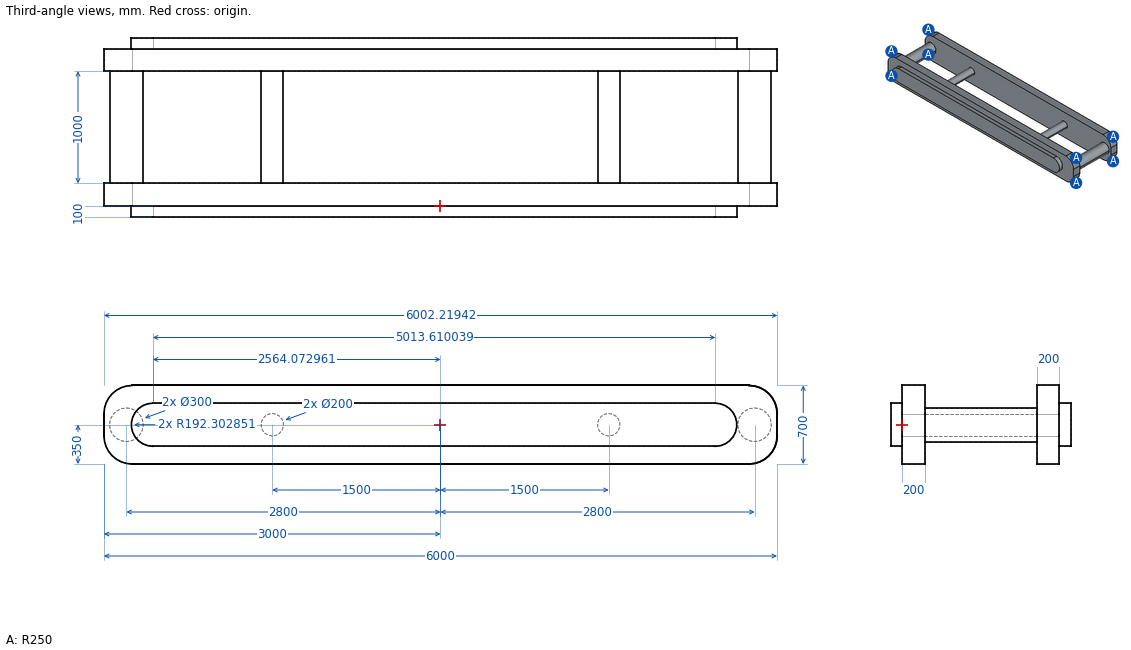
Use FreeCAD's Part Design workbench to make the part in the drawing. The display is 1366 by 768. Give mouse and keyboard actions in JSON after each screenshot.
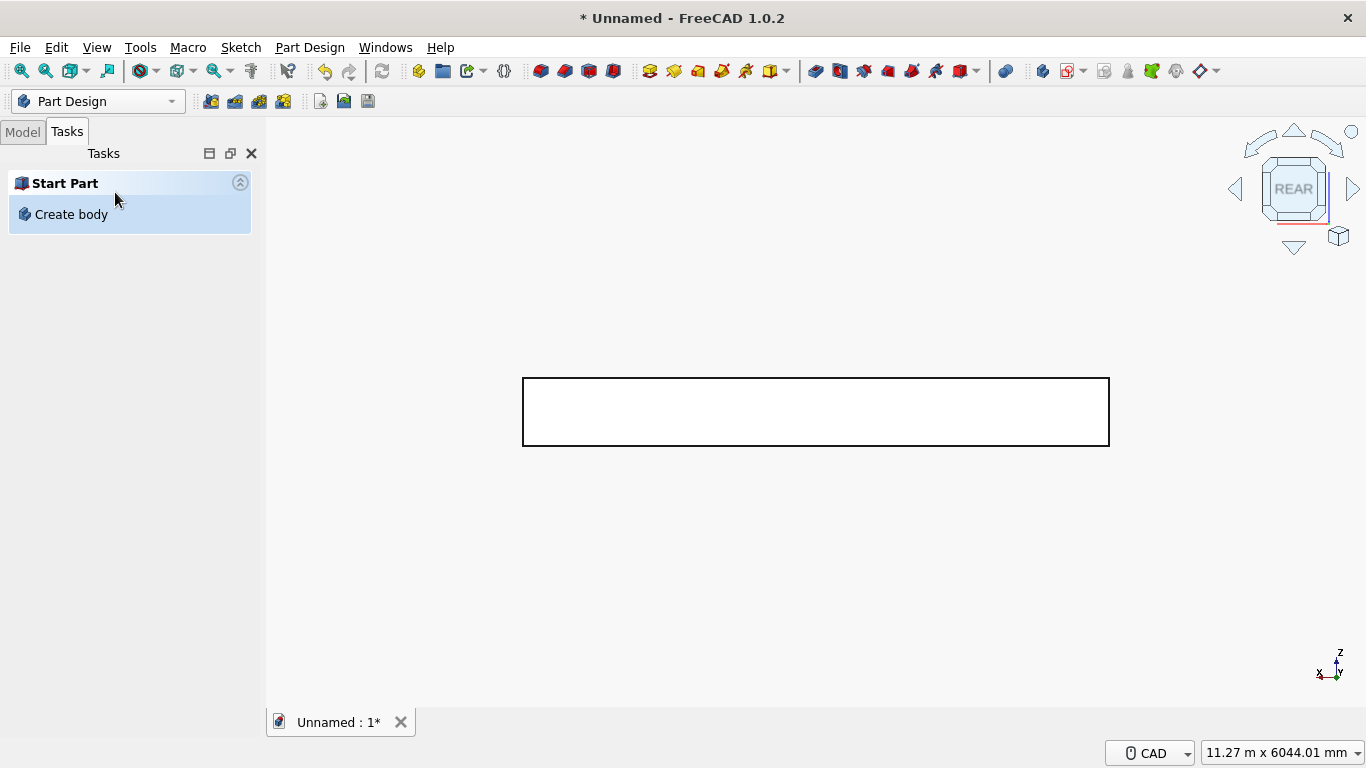
{"action": "scroll", "coordinate": [523, 445], "scroll_direction": "up", "scroll_amount": 4}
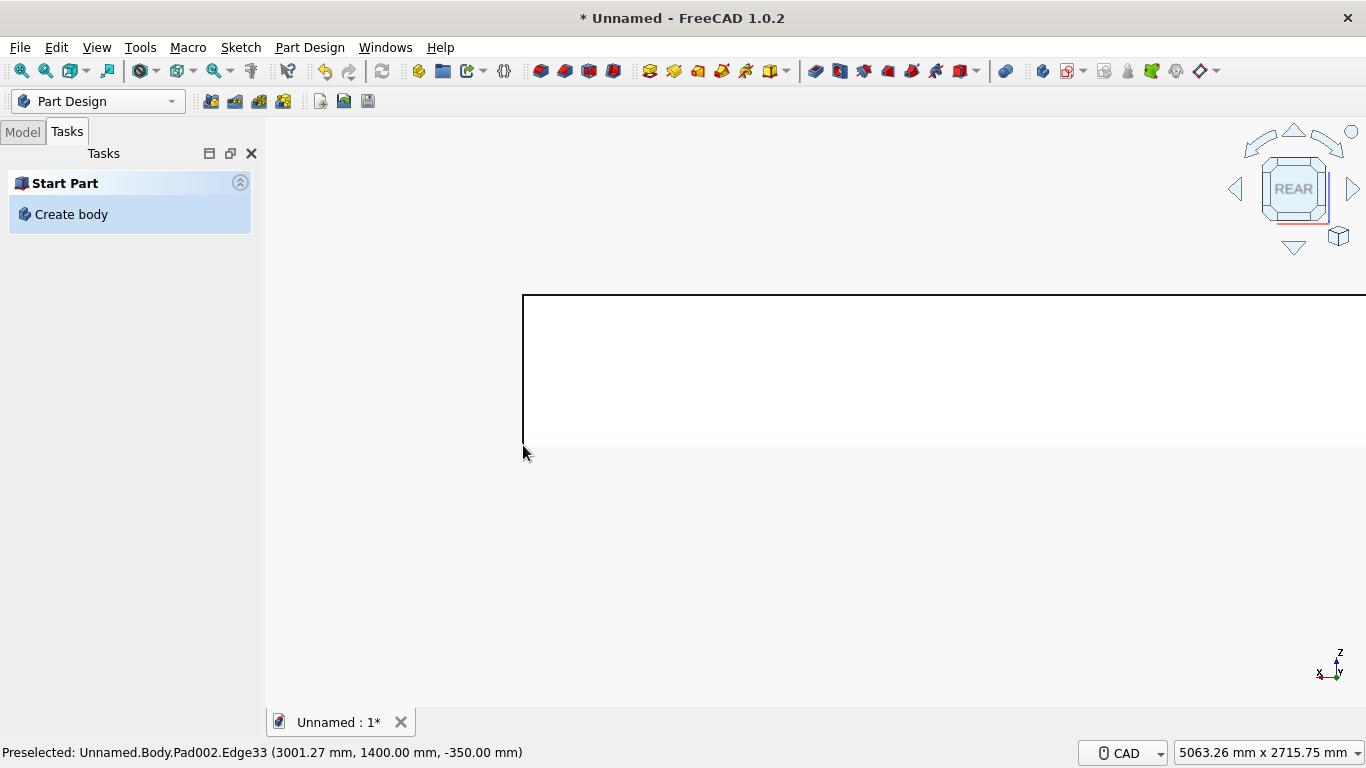
{"action": "left_click", "coordinate": [22, 72]}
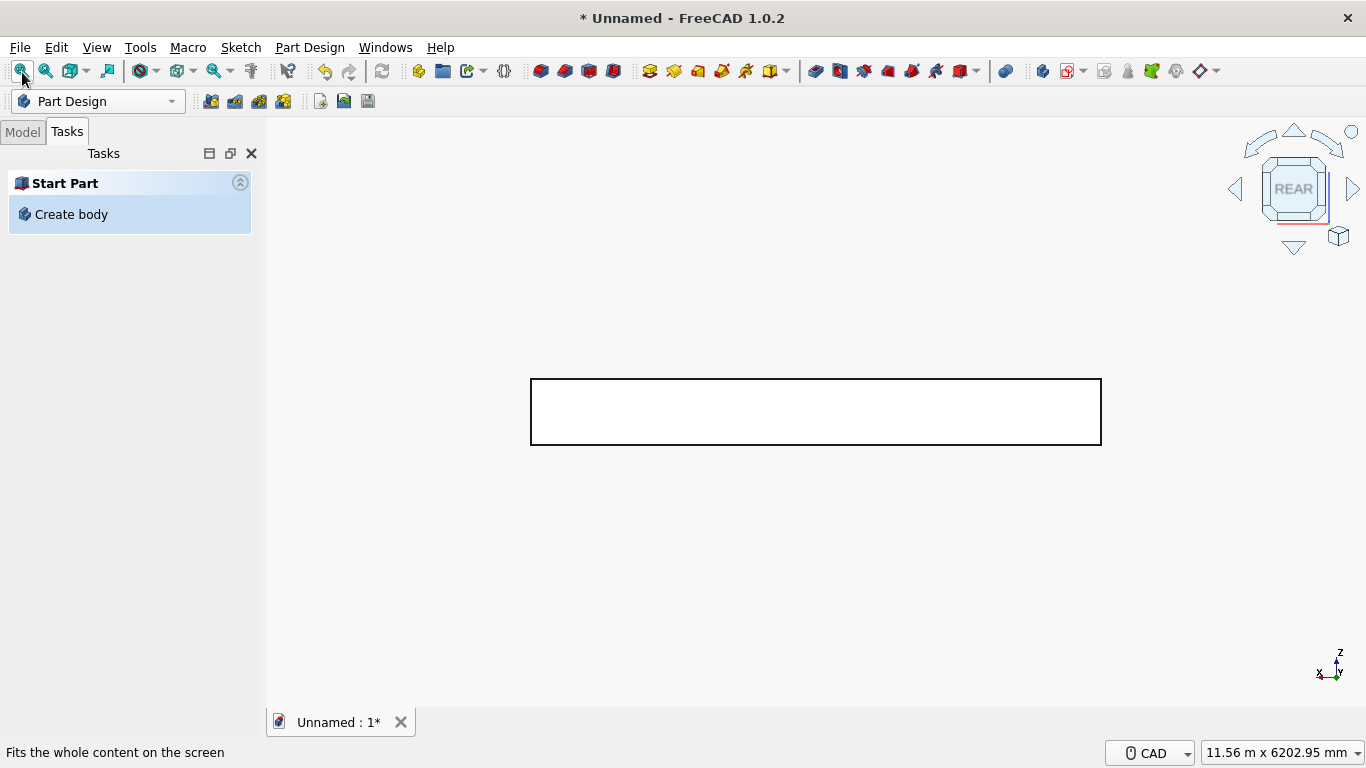
{"action": "key", "text": "0"}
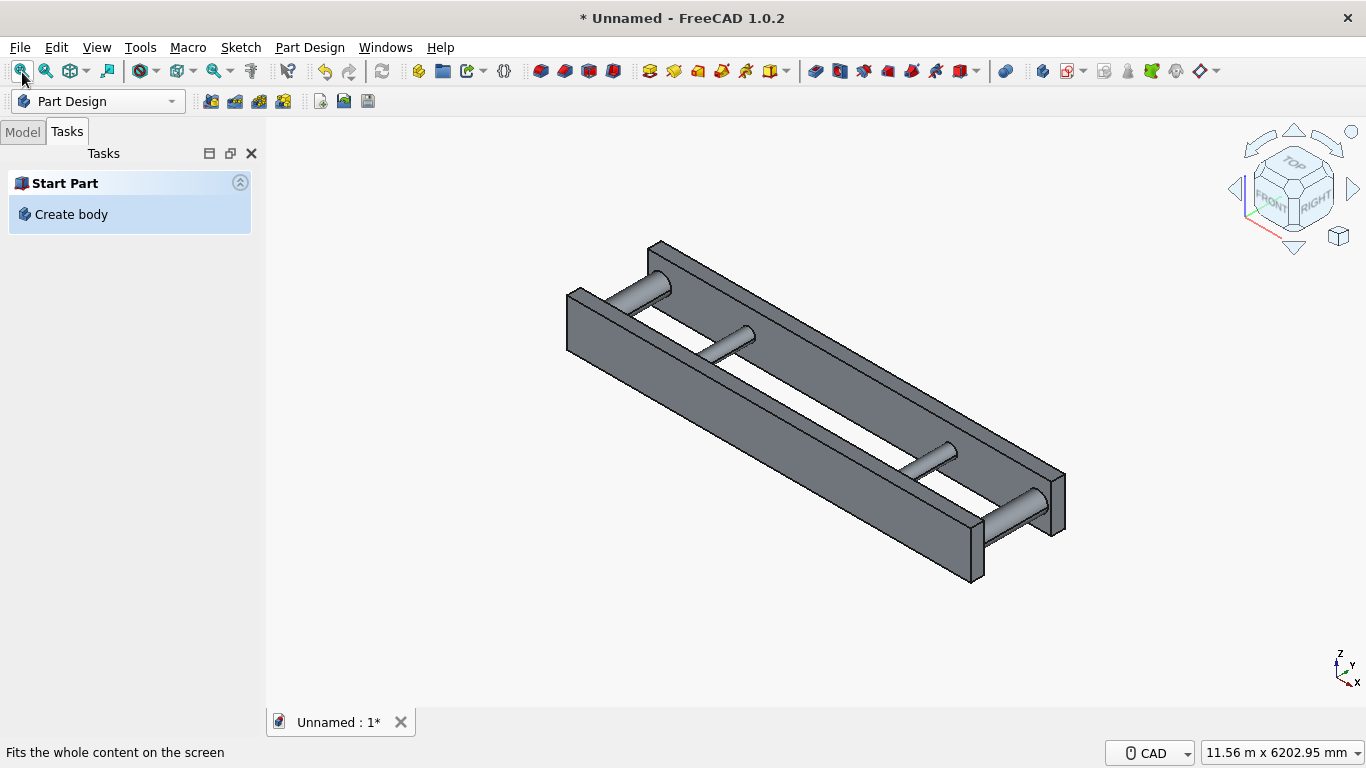
{"action": "left_click", "coordinate": [1058, 477]}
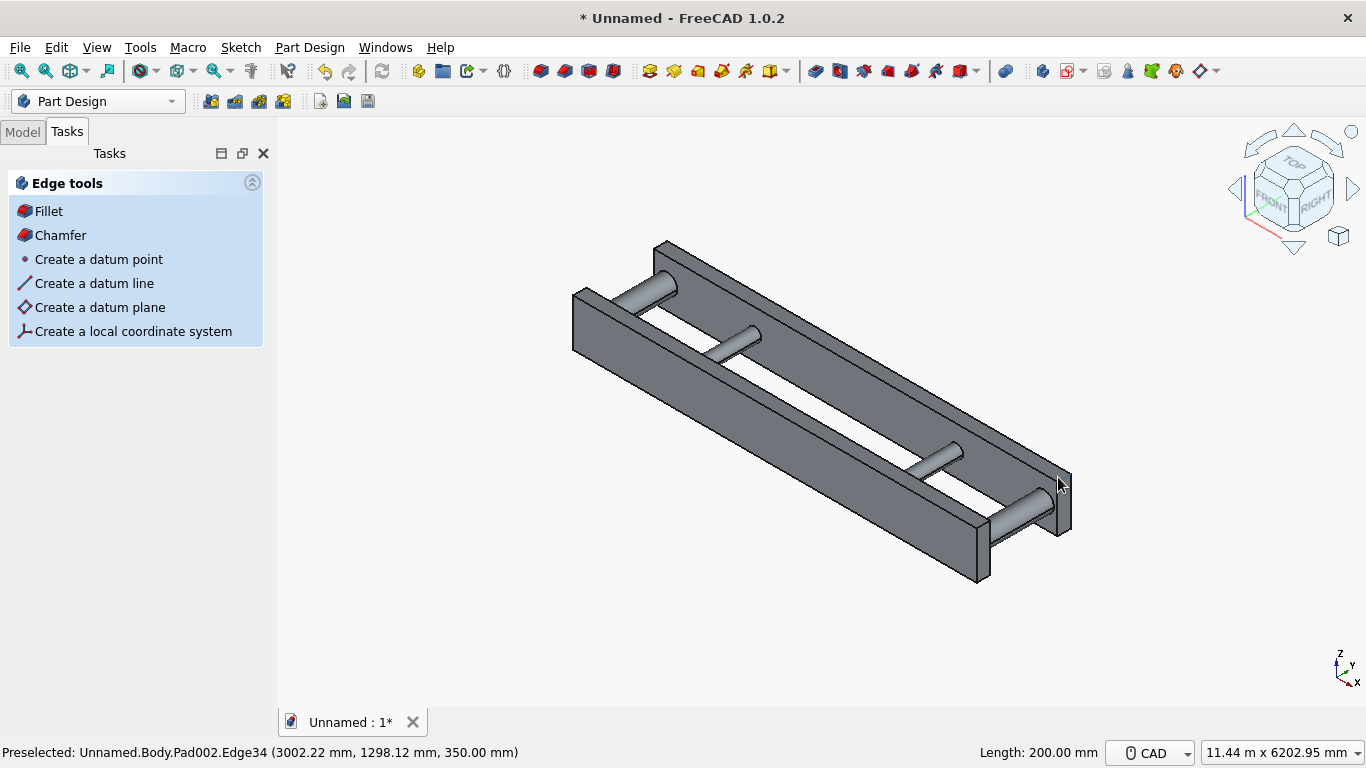
{"action": "left_click", "coordinate": [983, 524], "text": "ctrl"}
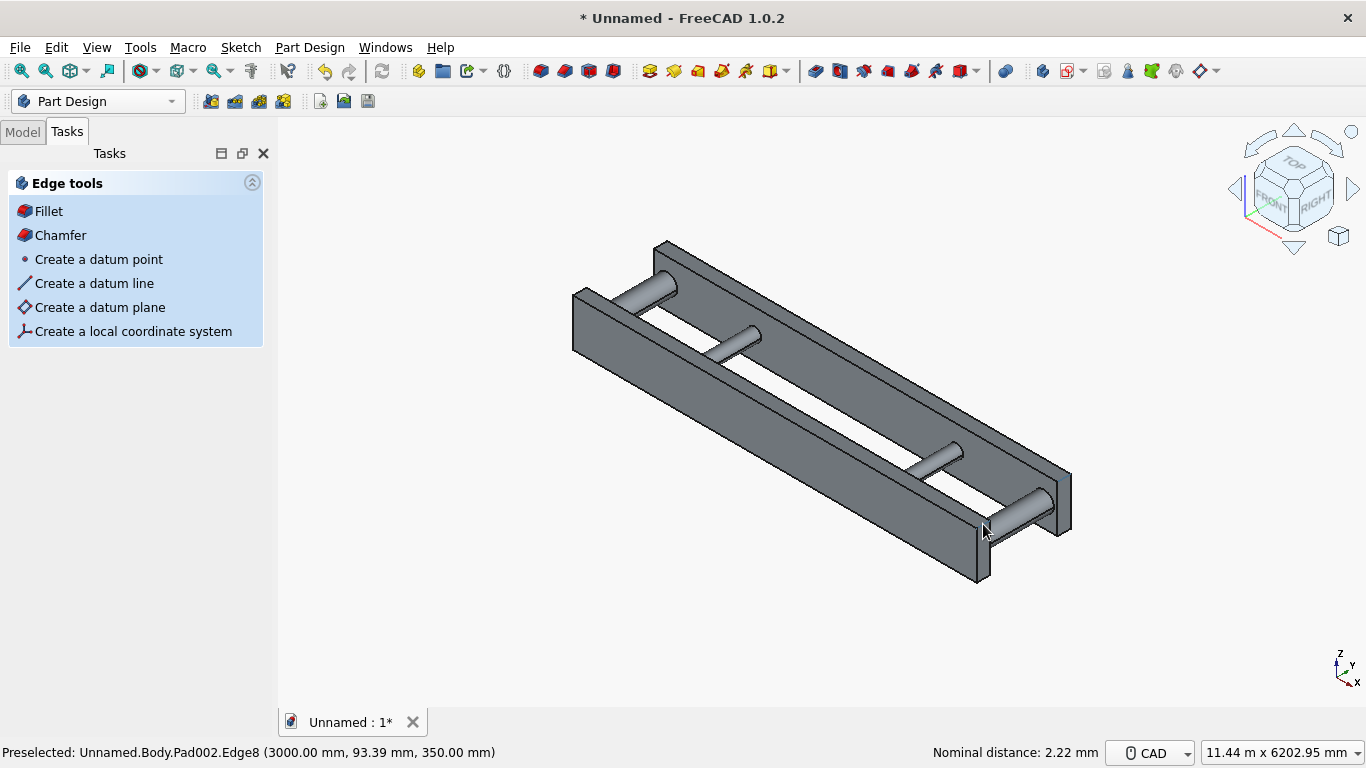
{"action": "scroll", "coordinate": [1064, 531], "scroll_direction": "up", "scroll_amount": 4}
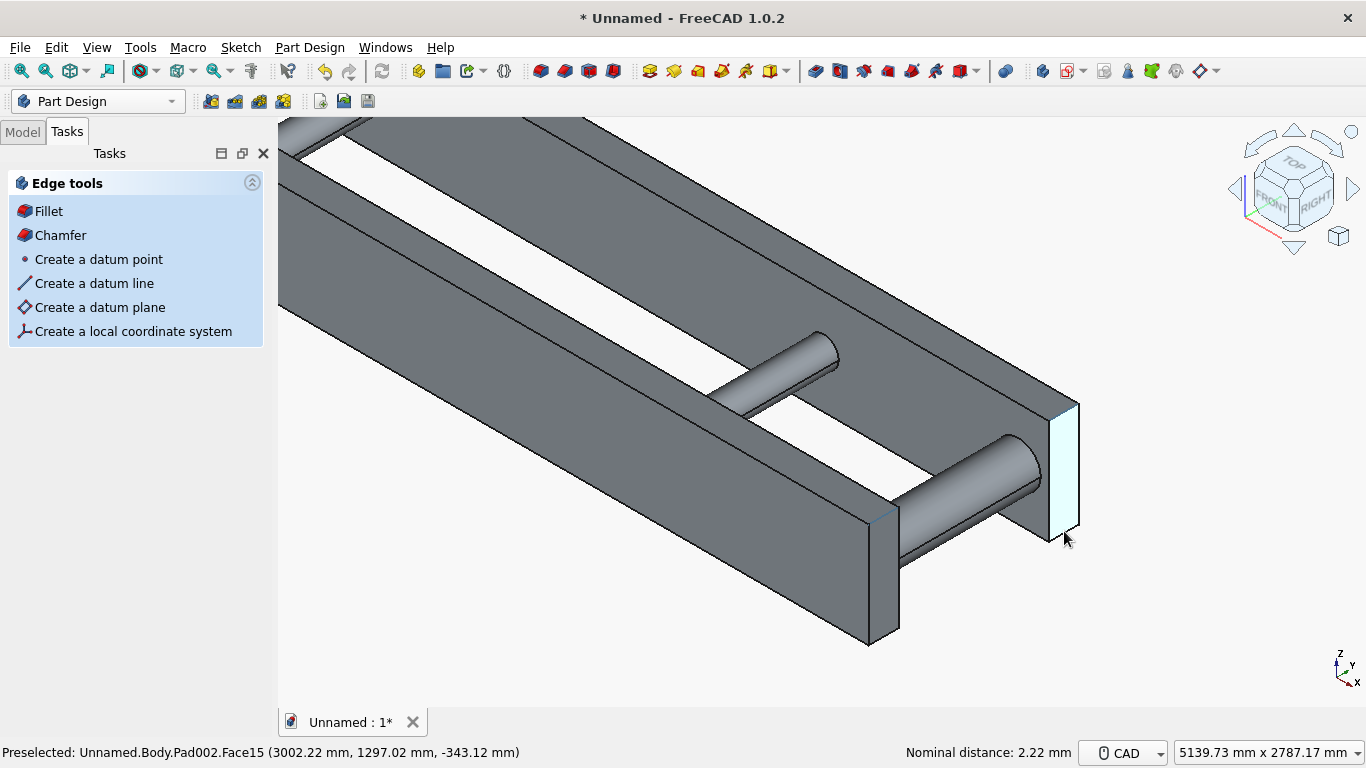
{"action": "left_click", "coordinate": [22, 72]}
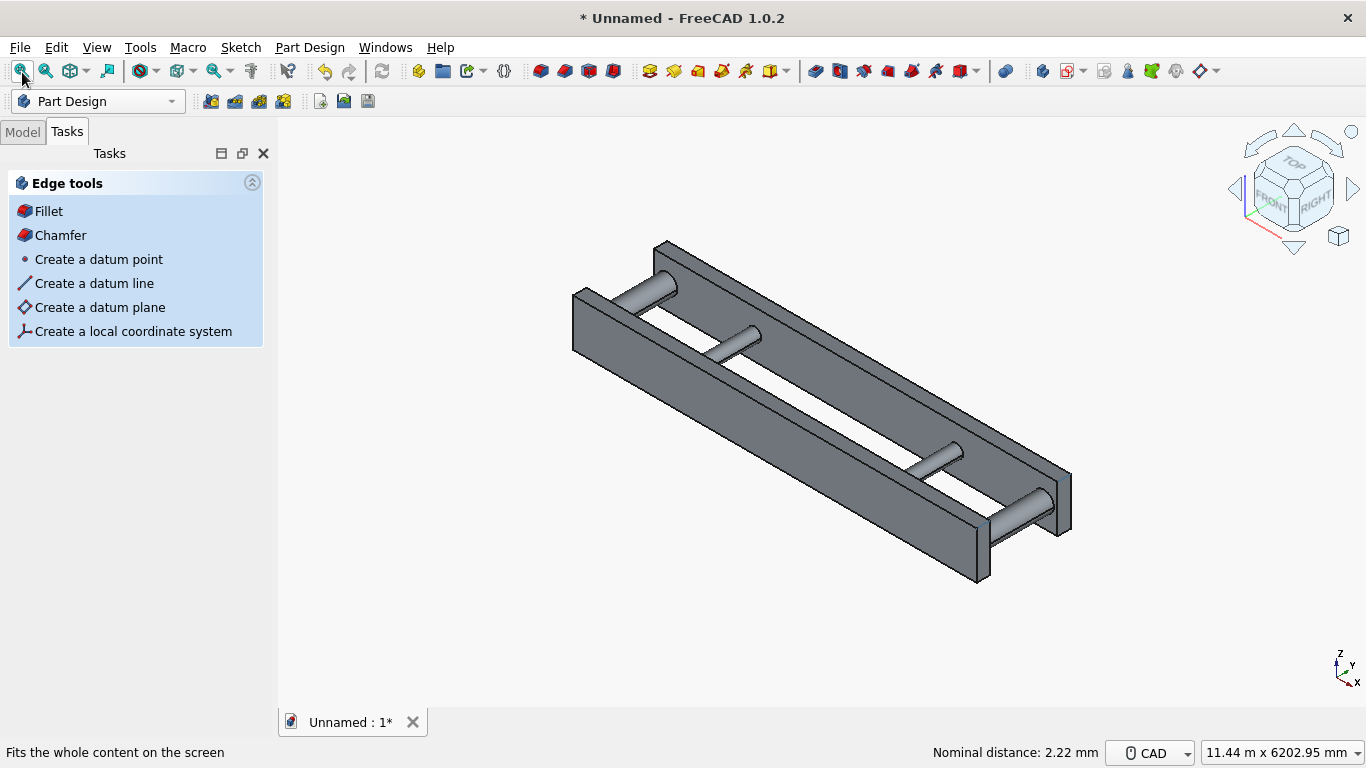
{"action": "key", "text": "2"}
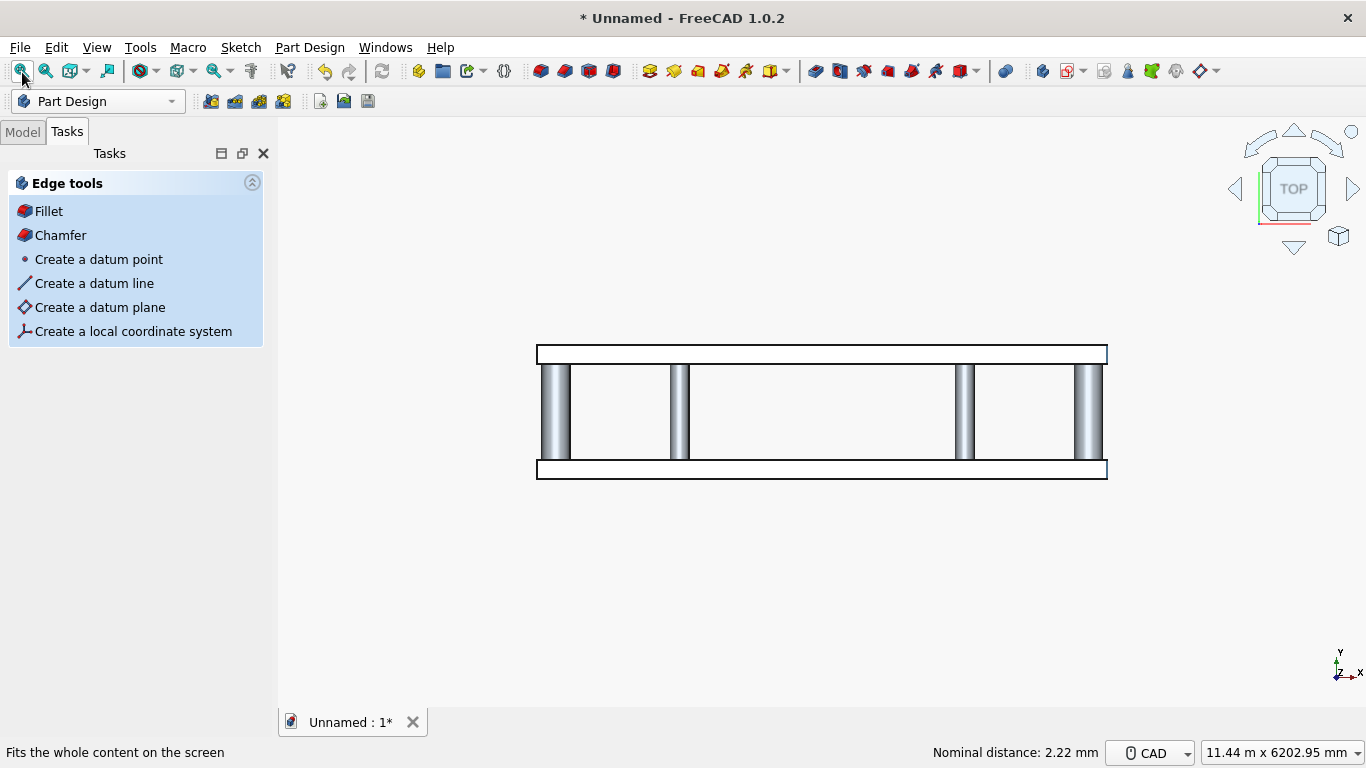
{"action": "left_click", "coordinate": [537, 354], "text": "ctrl"}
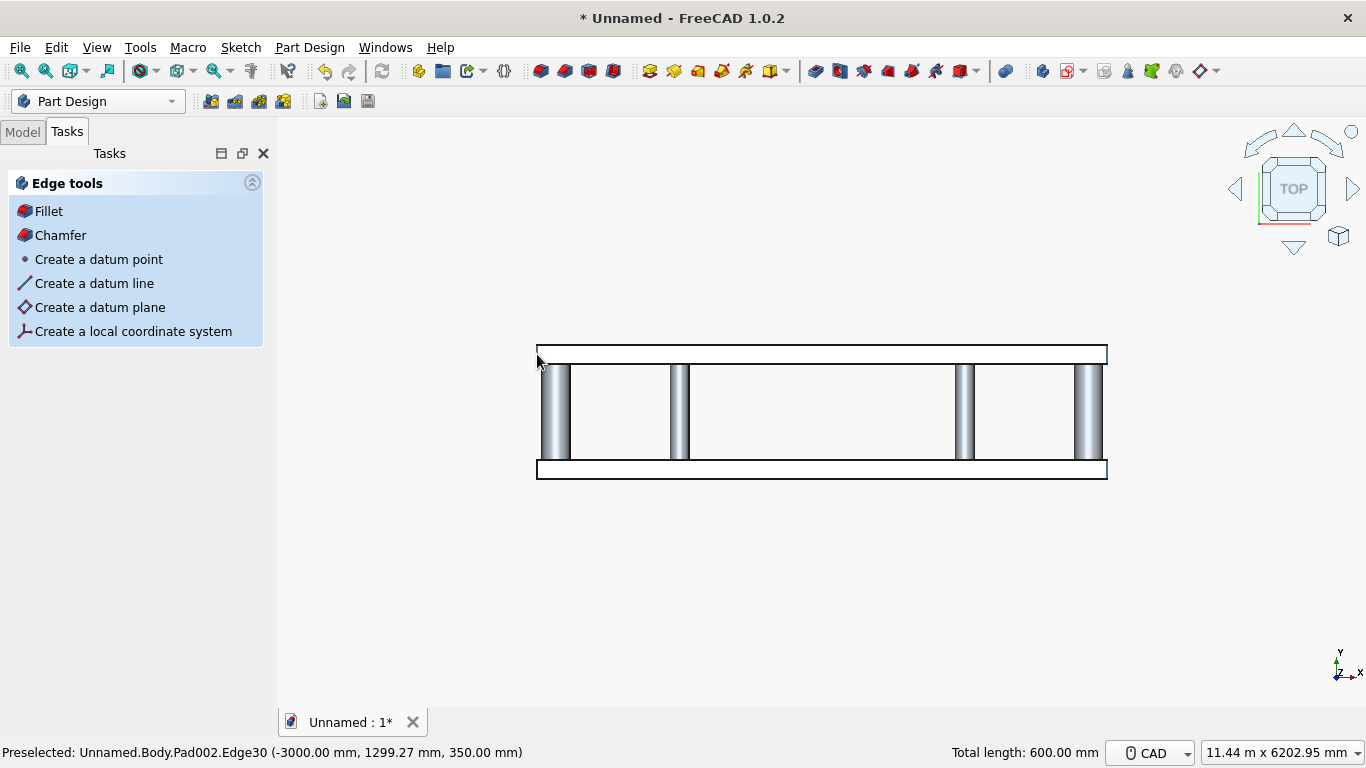
{"action": "left_click", "coordinate": [537, 468], "text": "ctrl"}